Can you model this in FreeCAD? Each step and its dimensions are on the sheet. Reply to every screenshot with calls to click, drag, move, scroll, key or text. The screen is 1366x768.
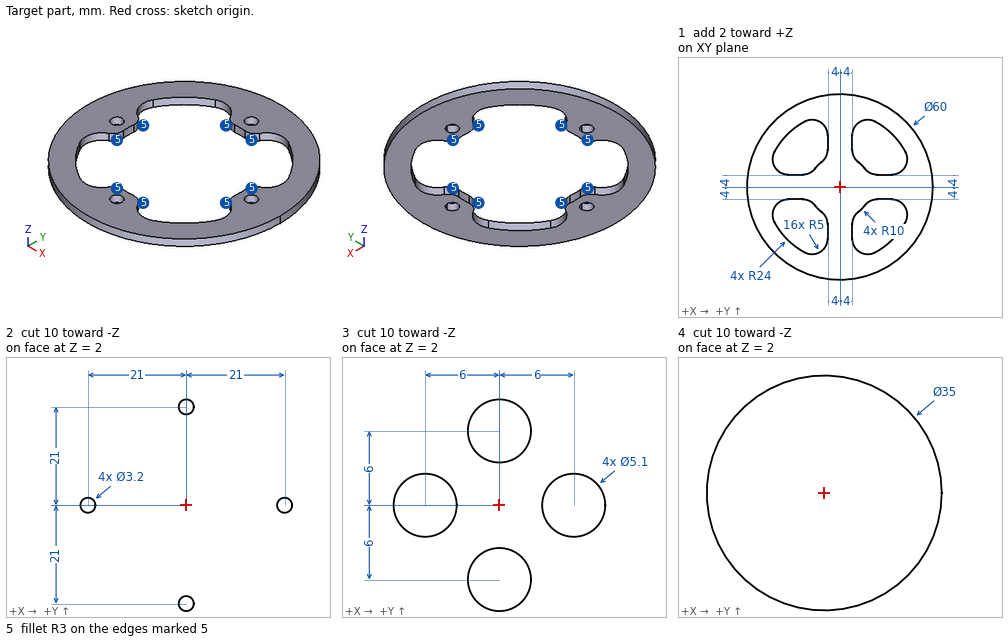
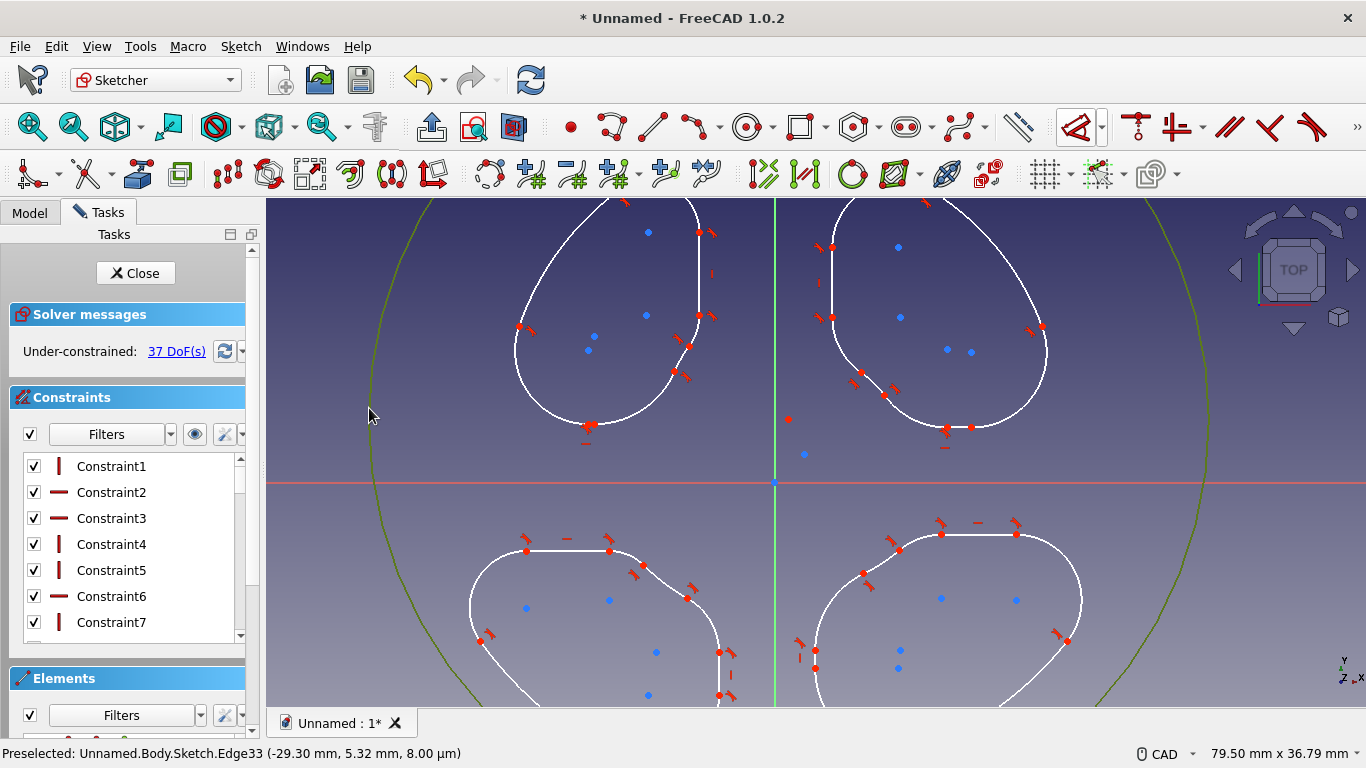
scroll(879, 388, up, 2)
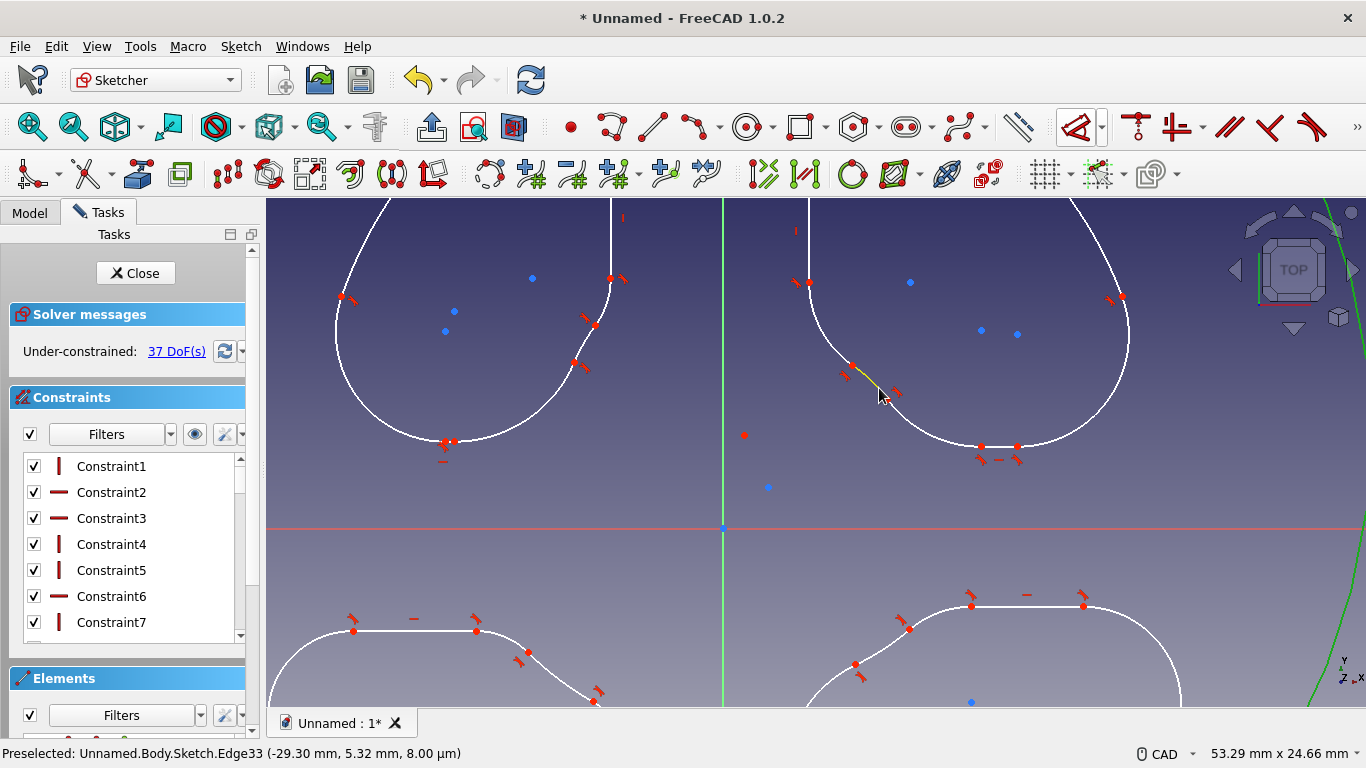
click(878, 388)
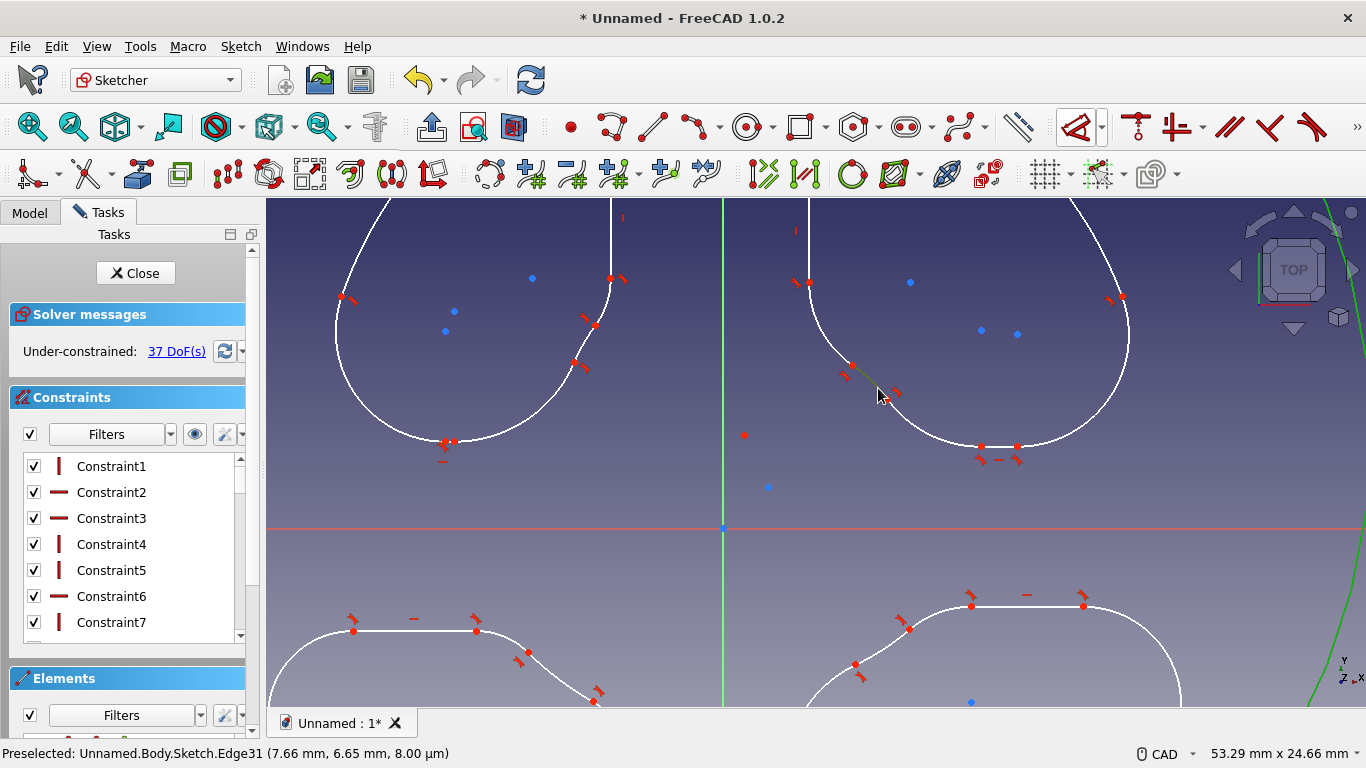
key(c)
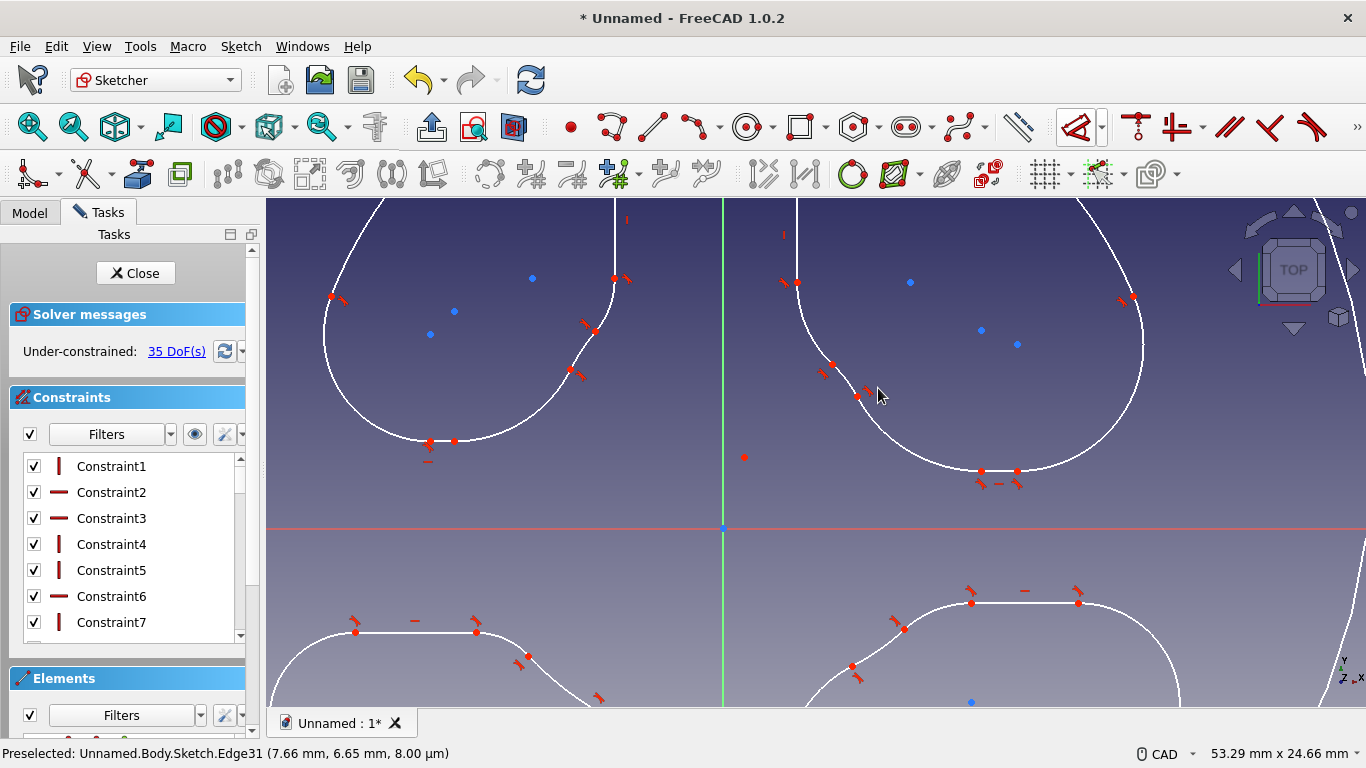
drag(713, 447, 755, 539)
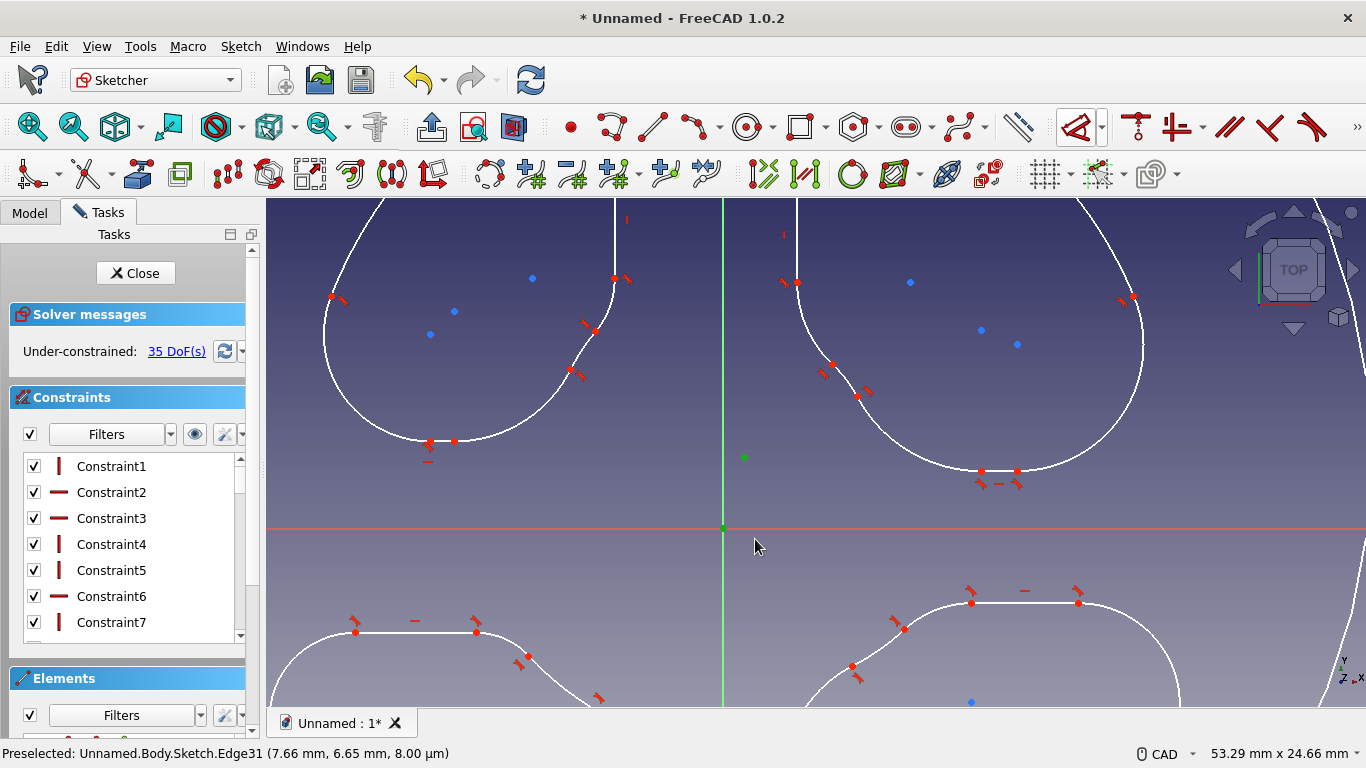
key(c)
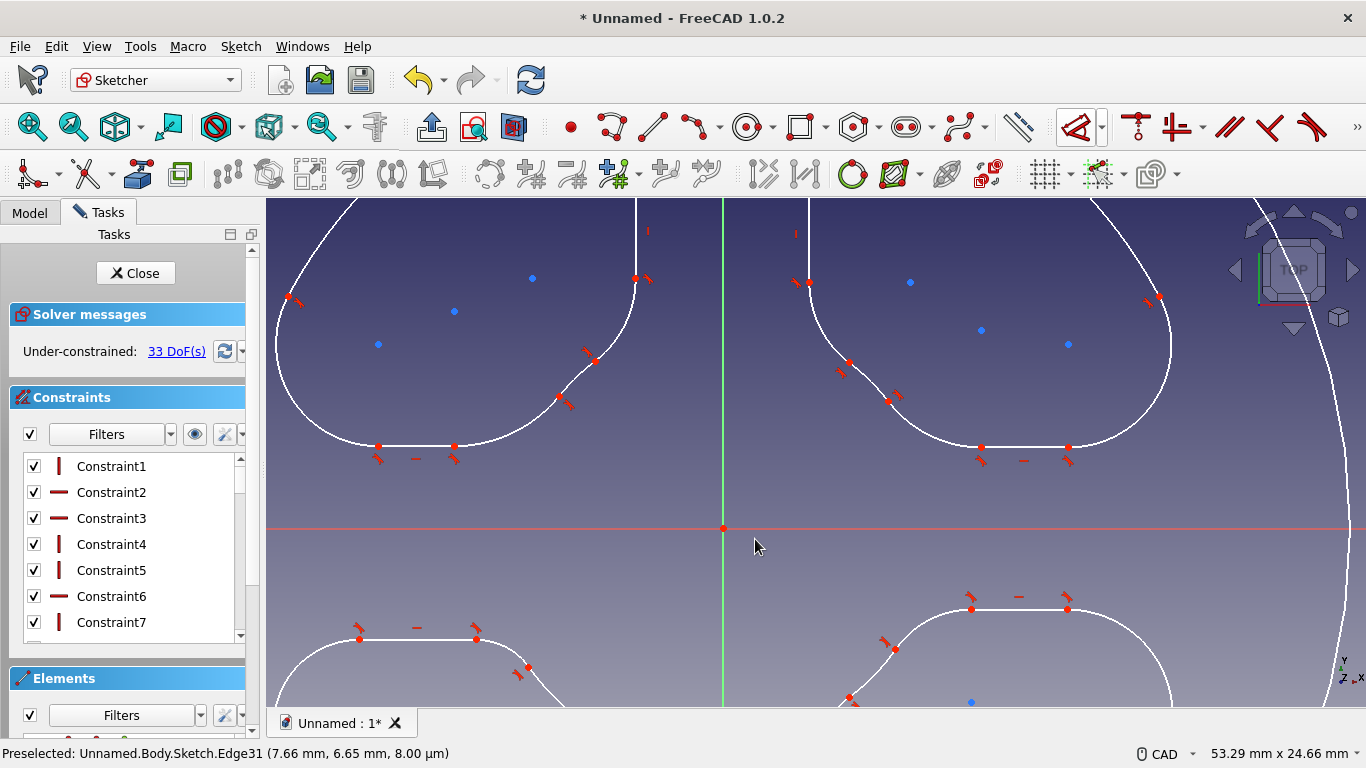
scroll(755, 427, down, 7)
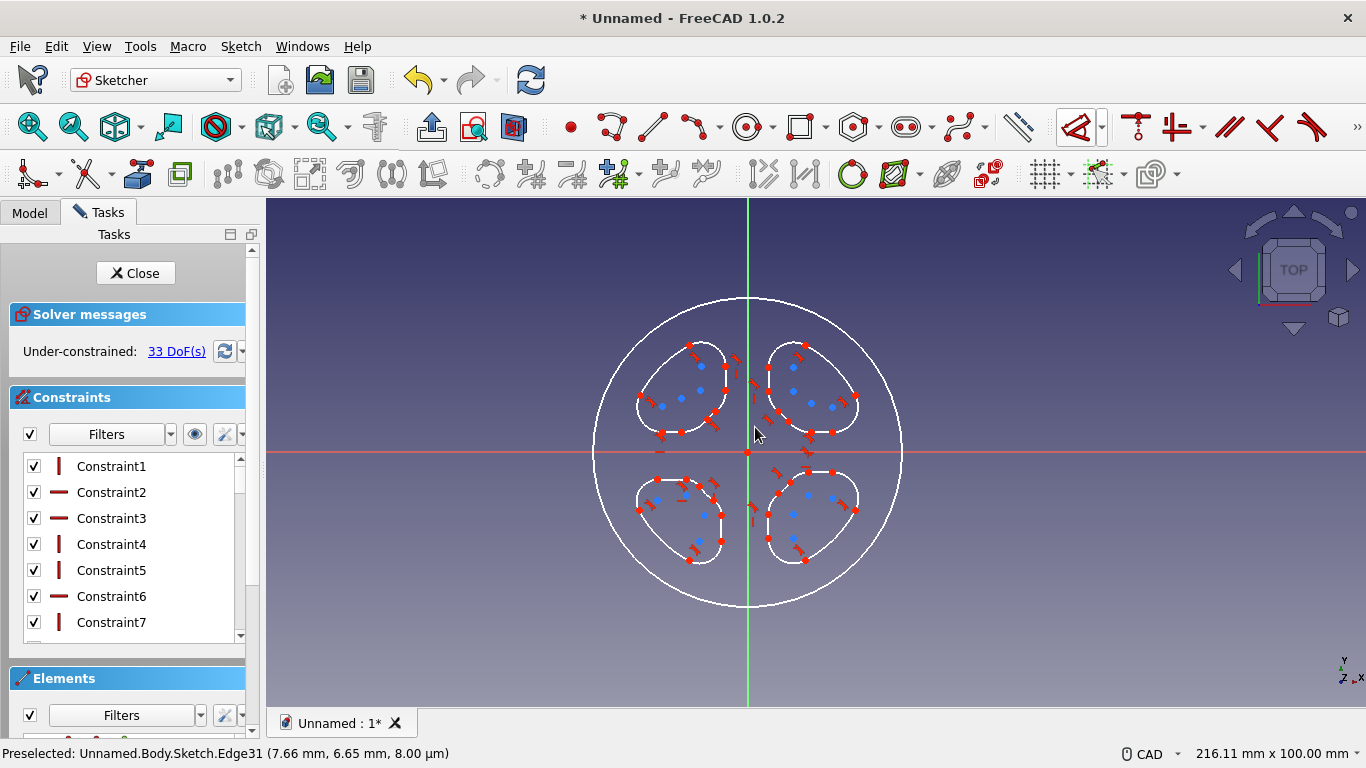
click(702, 563)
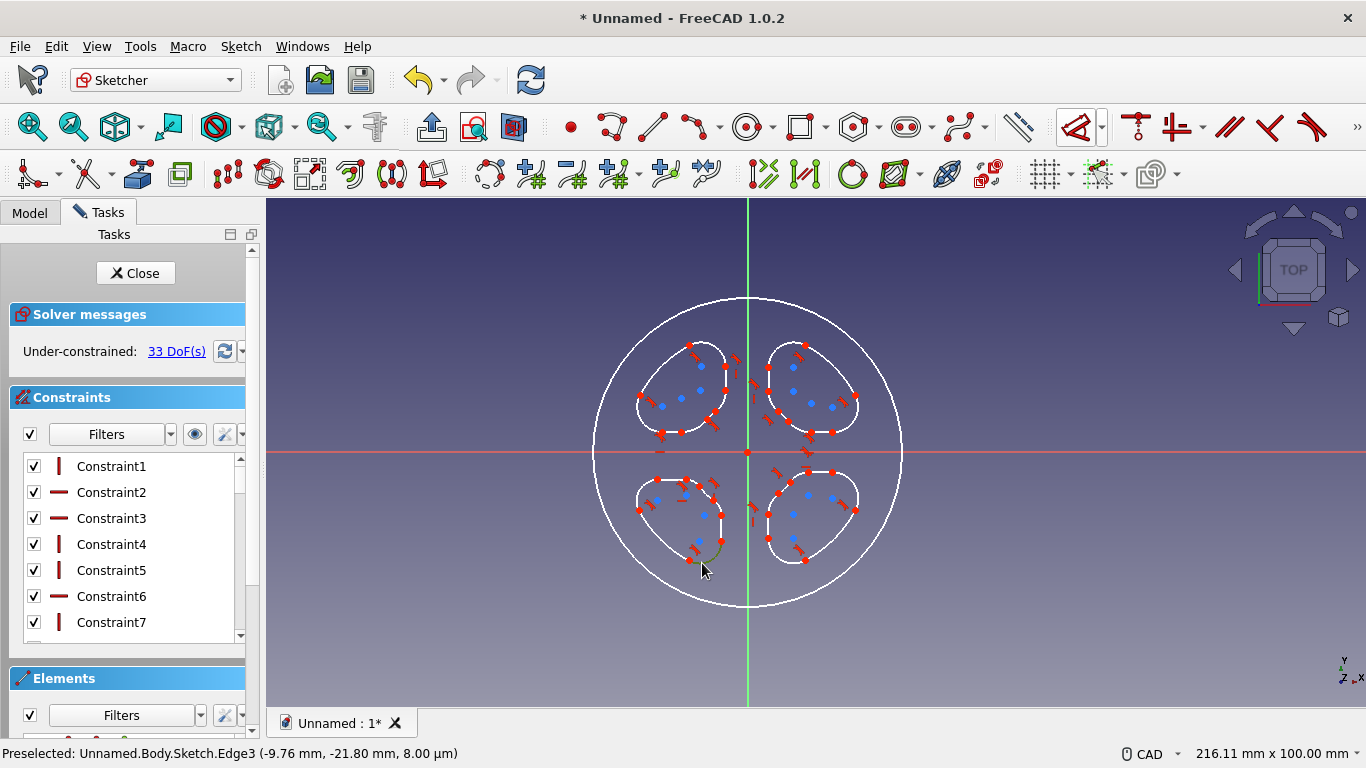
click(646, 484)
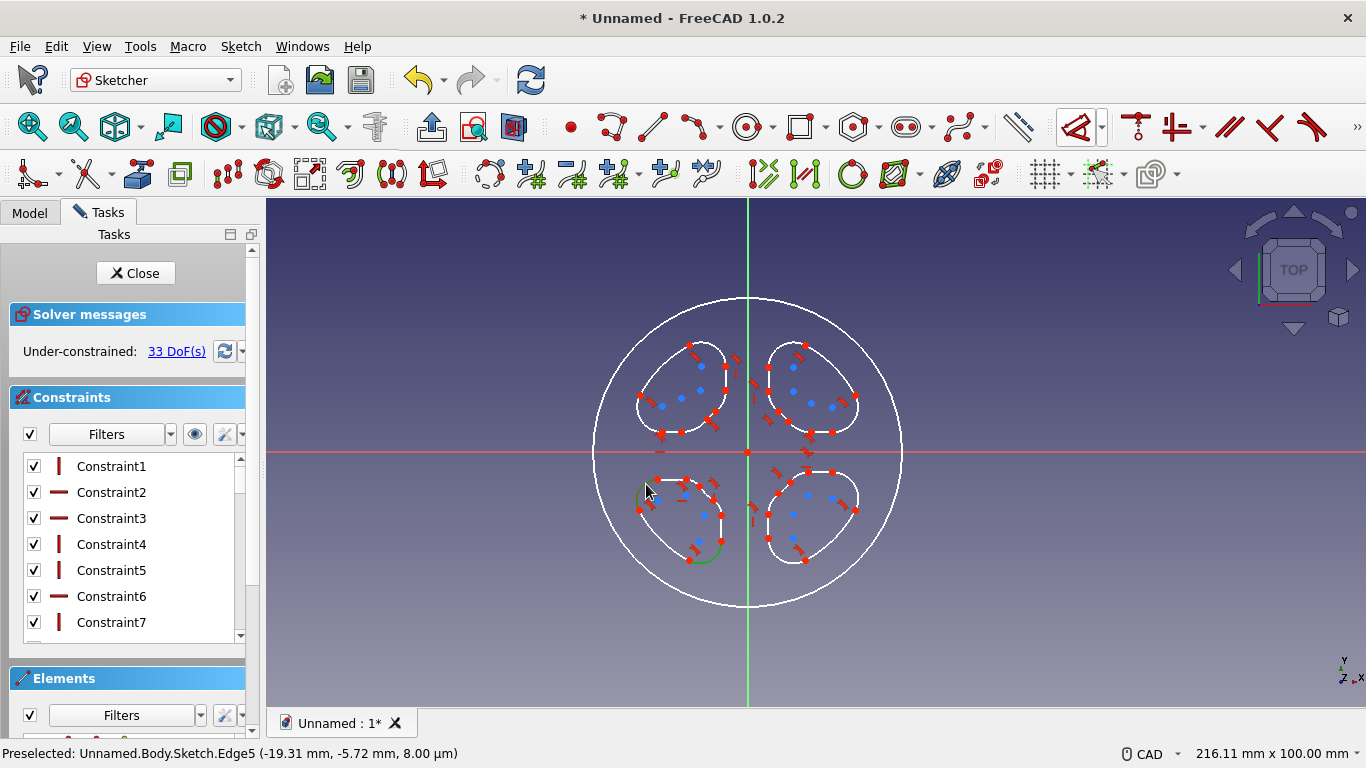
scroll(694, 482, up, 4)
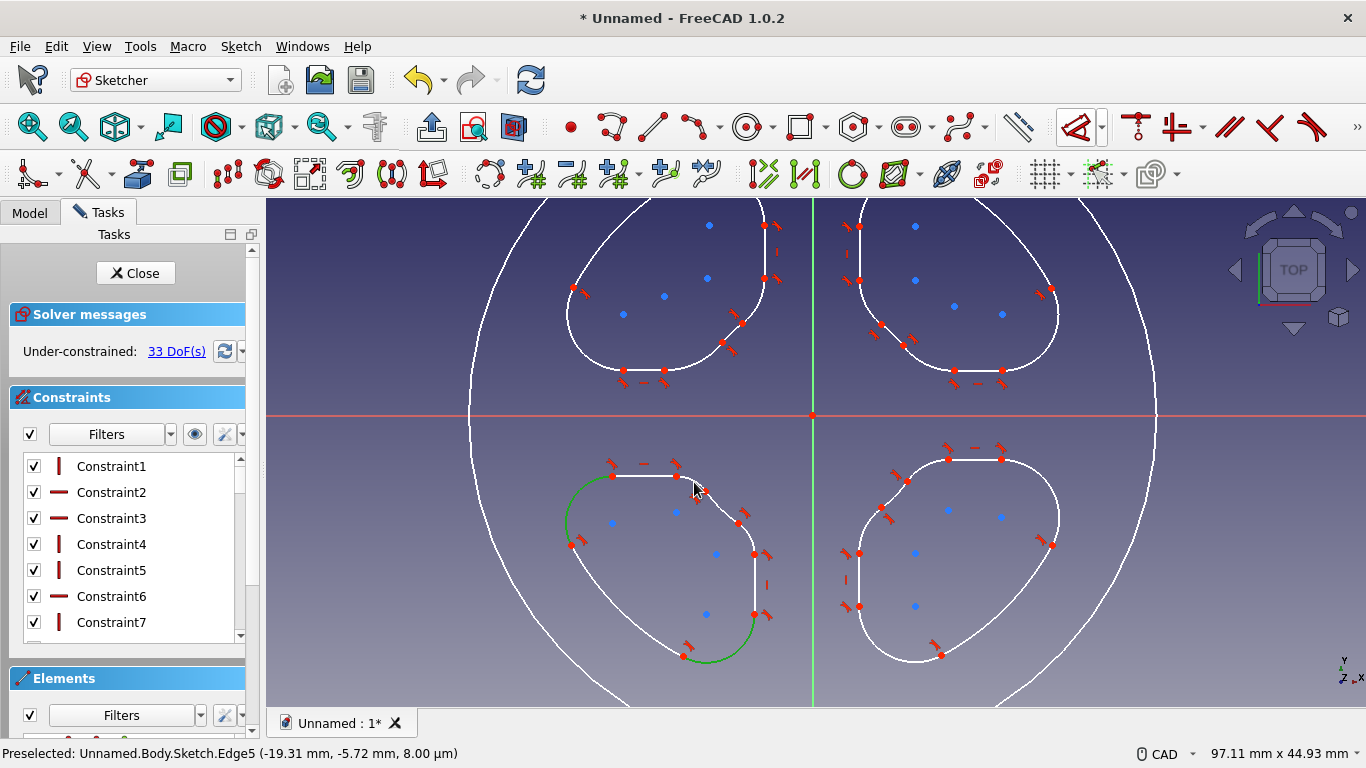
click(693, 480)